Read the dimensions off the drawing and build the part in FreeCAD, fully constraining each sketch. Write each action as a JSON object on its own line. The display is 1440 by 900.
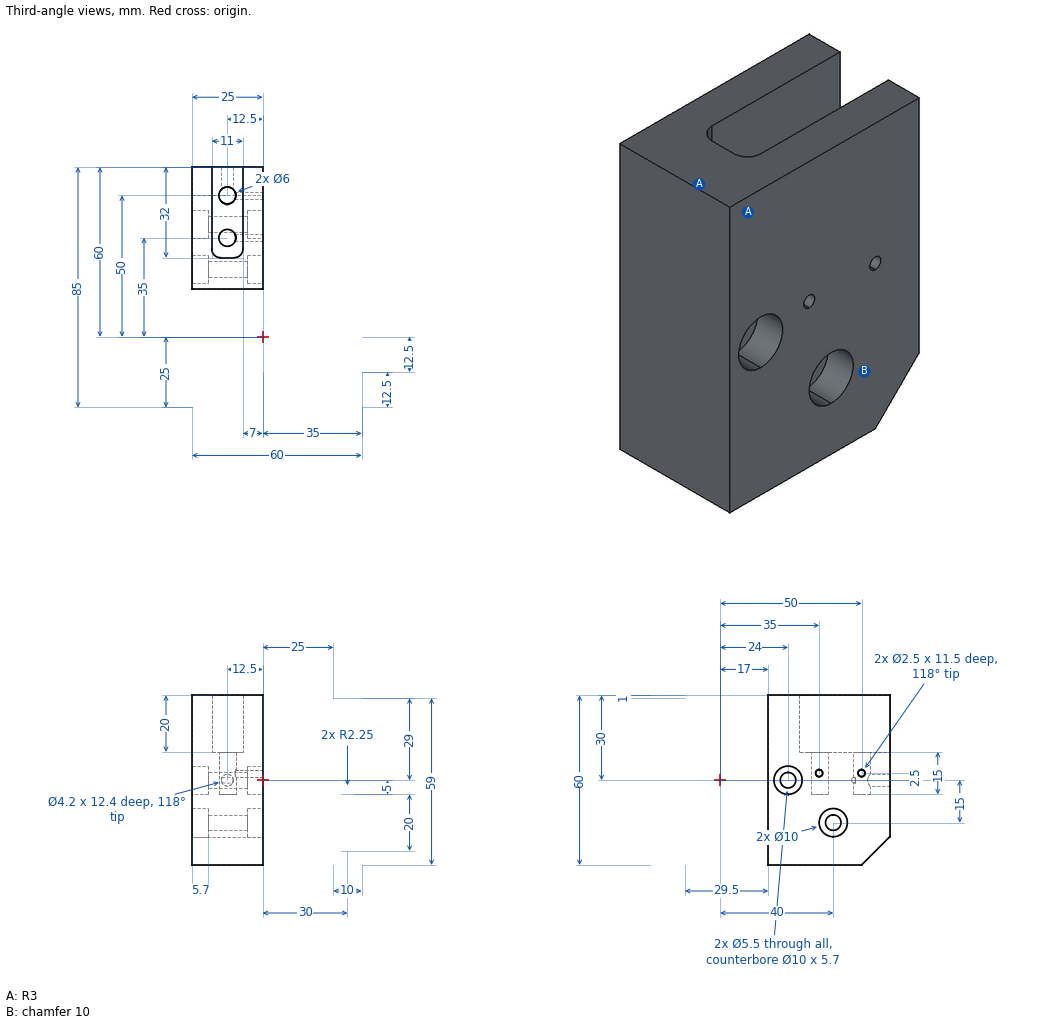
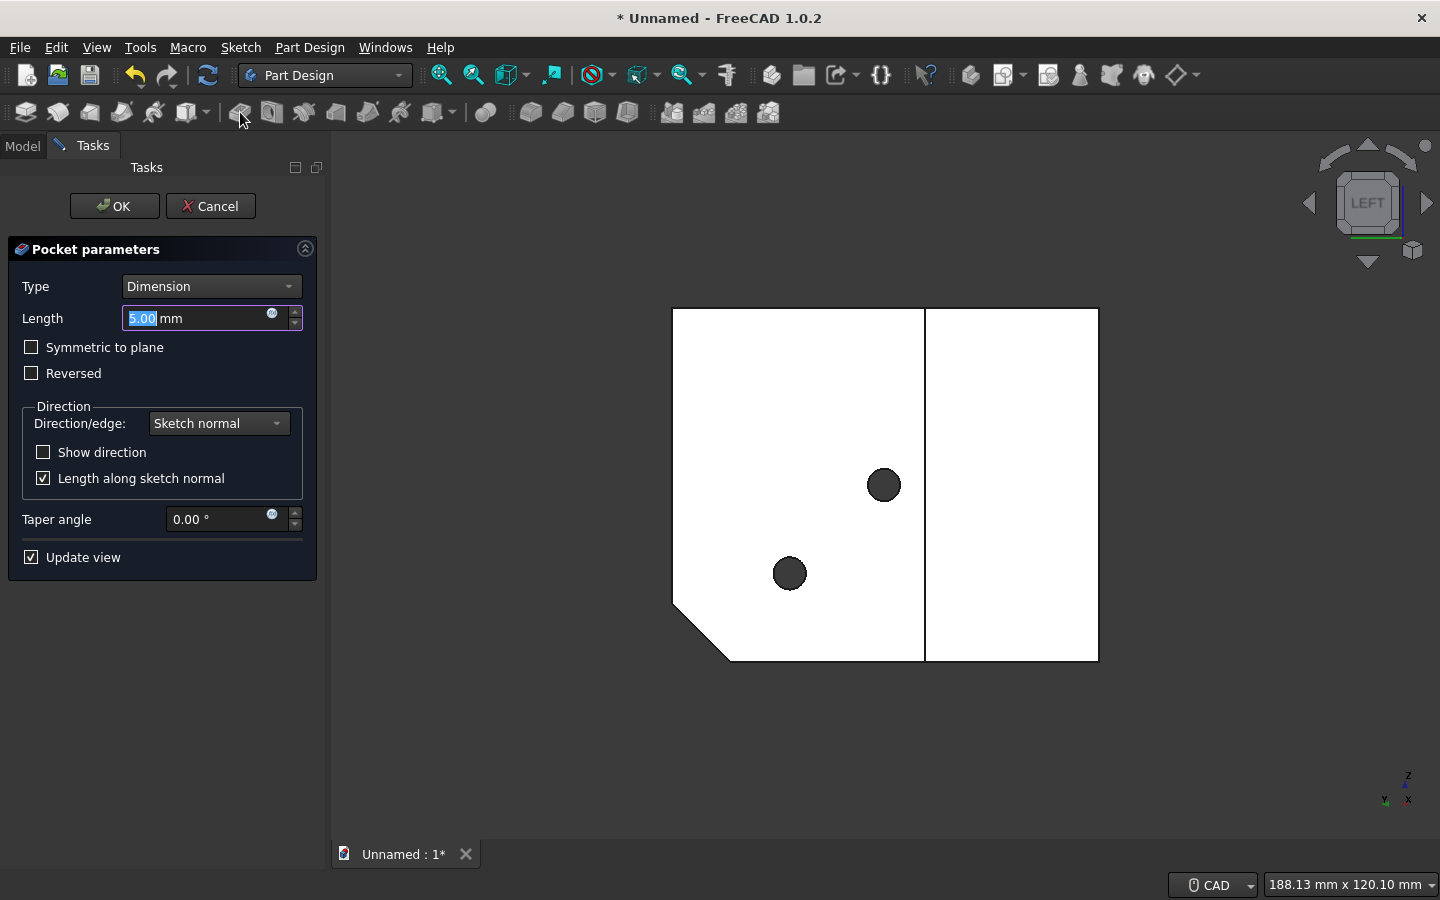
{"action": "left_click", "coordinate": [212, 286]}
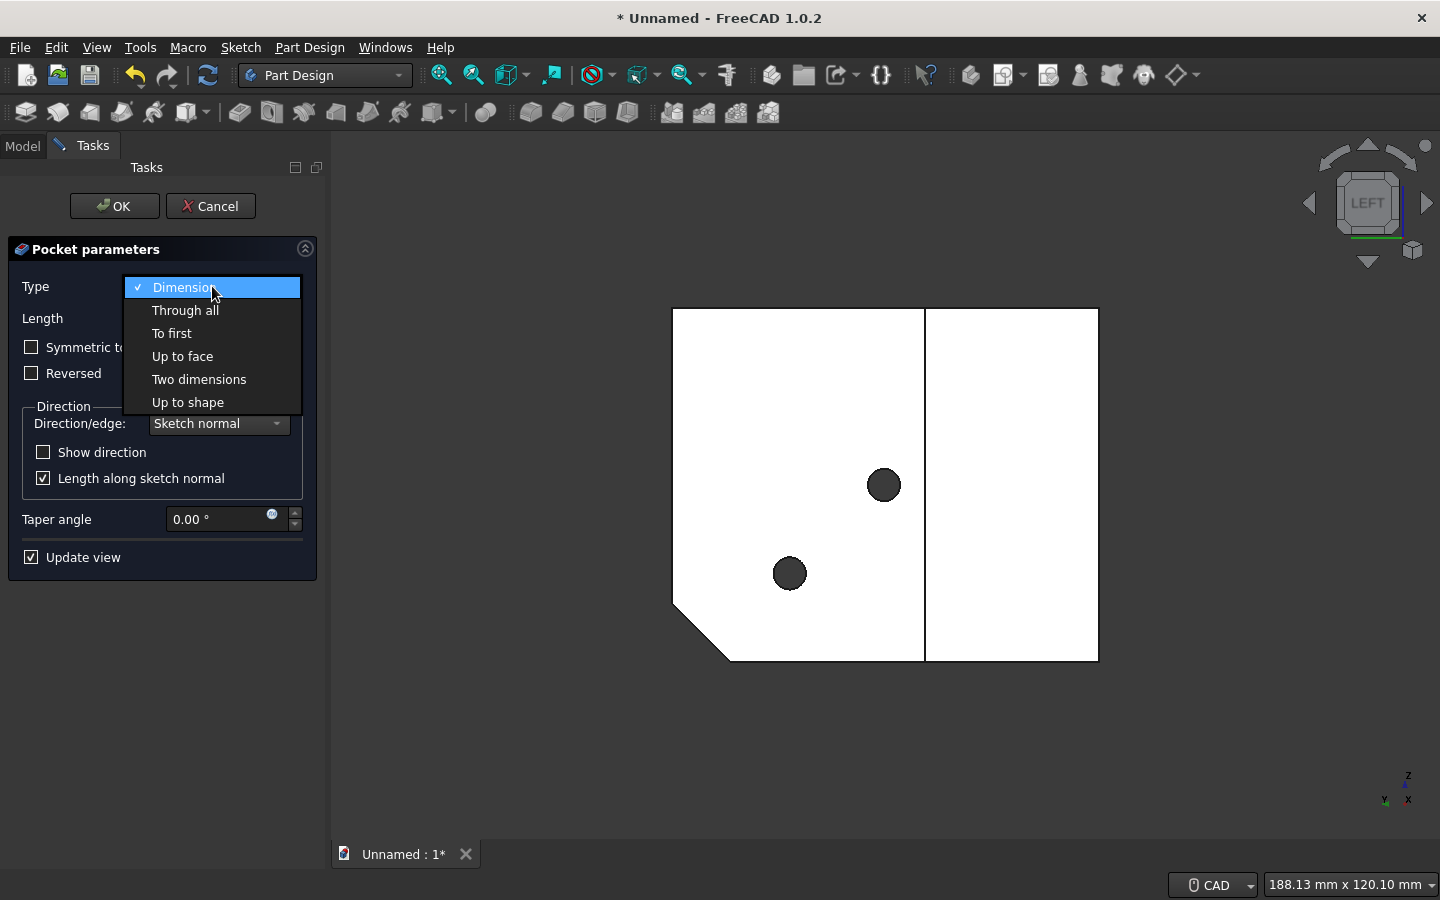
{"action": "left_click", "coordinate": [212, 310]}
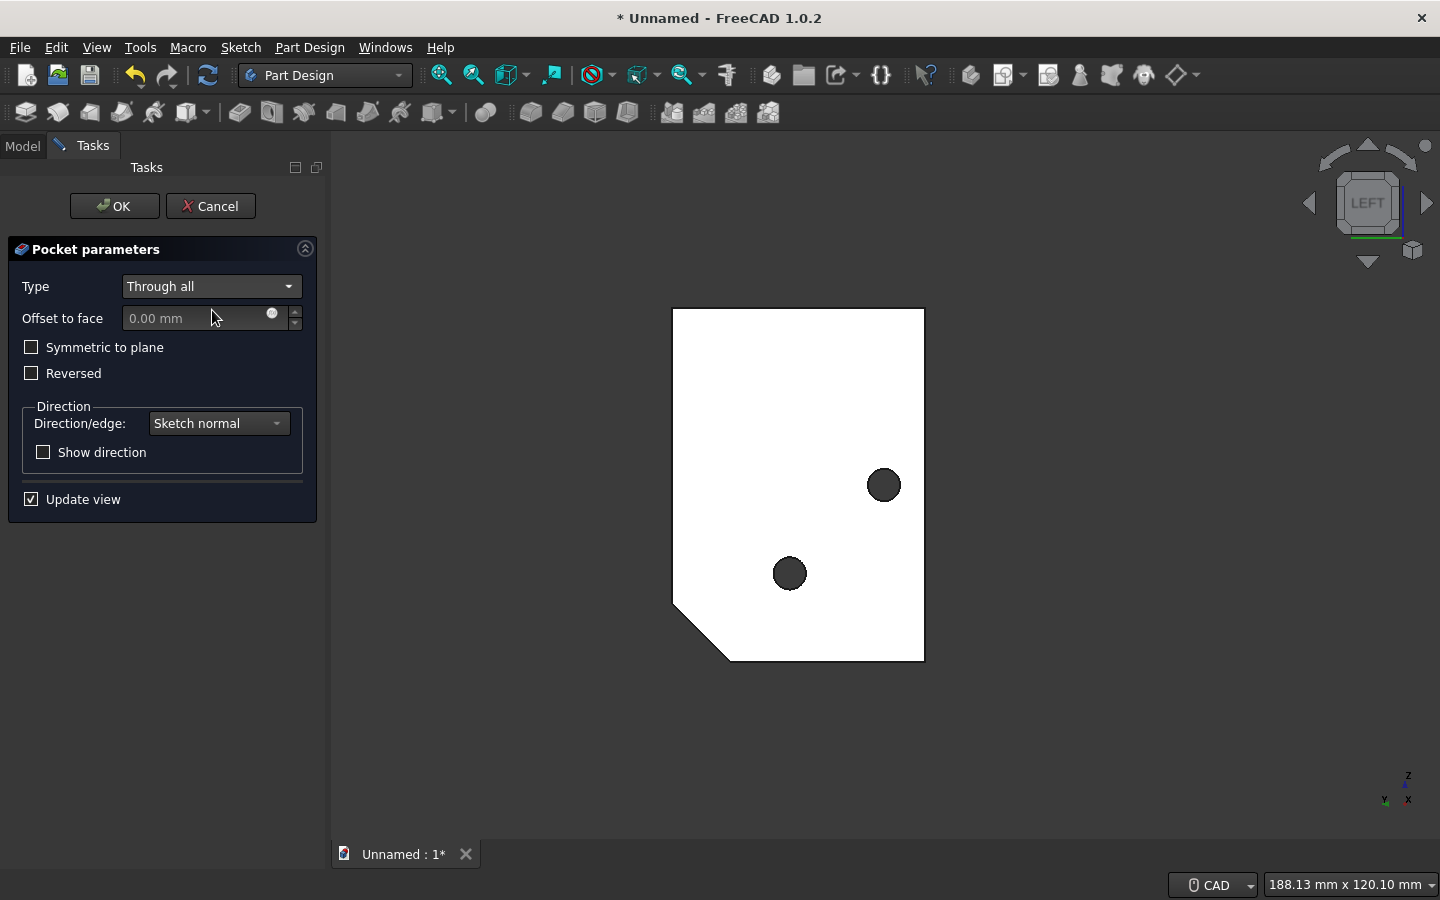
{"action": "left_click", "coordinate": [115, 206]}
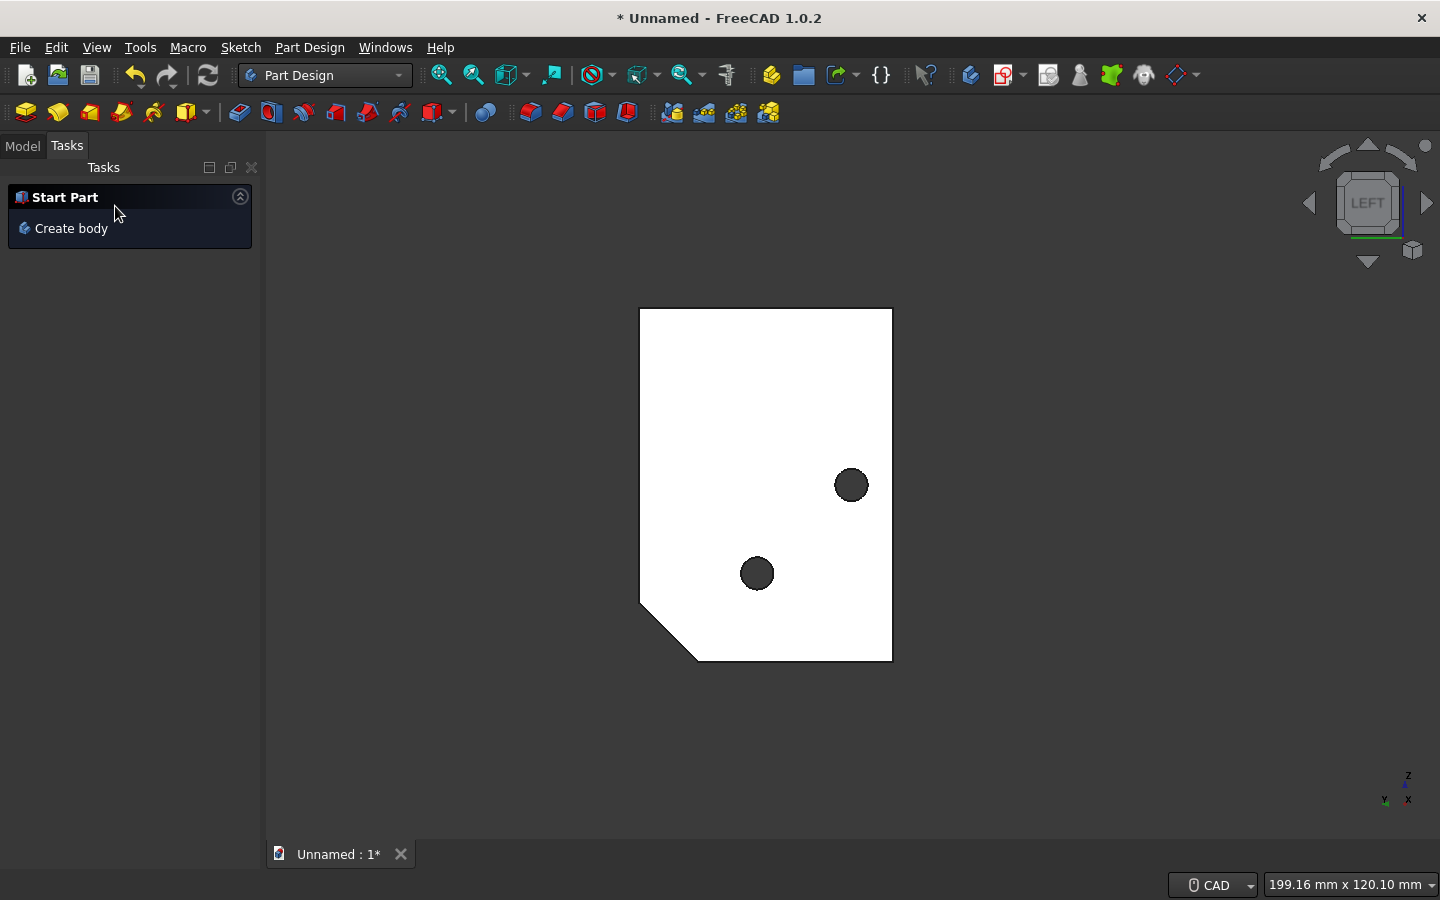
{"action": "left_click", "coordinate": [23, 145]}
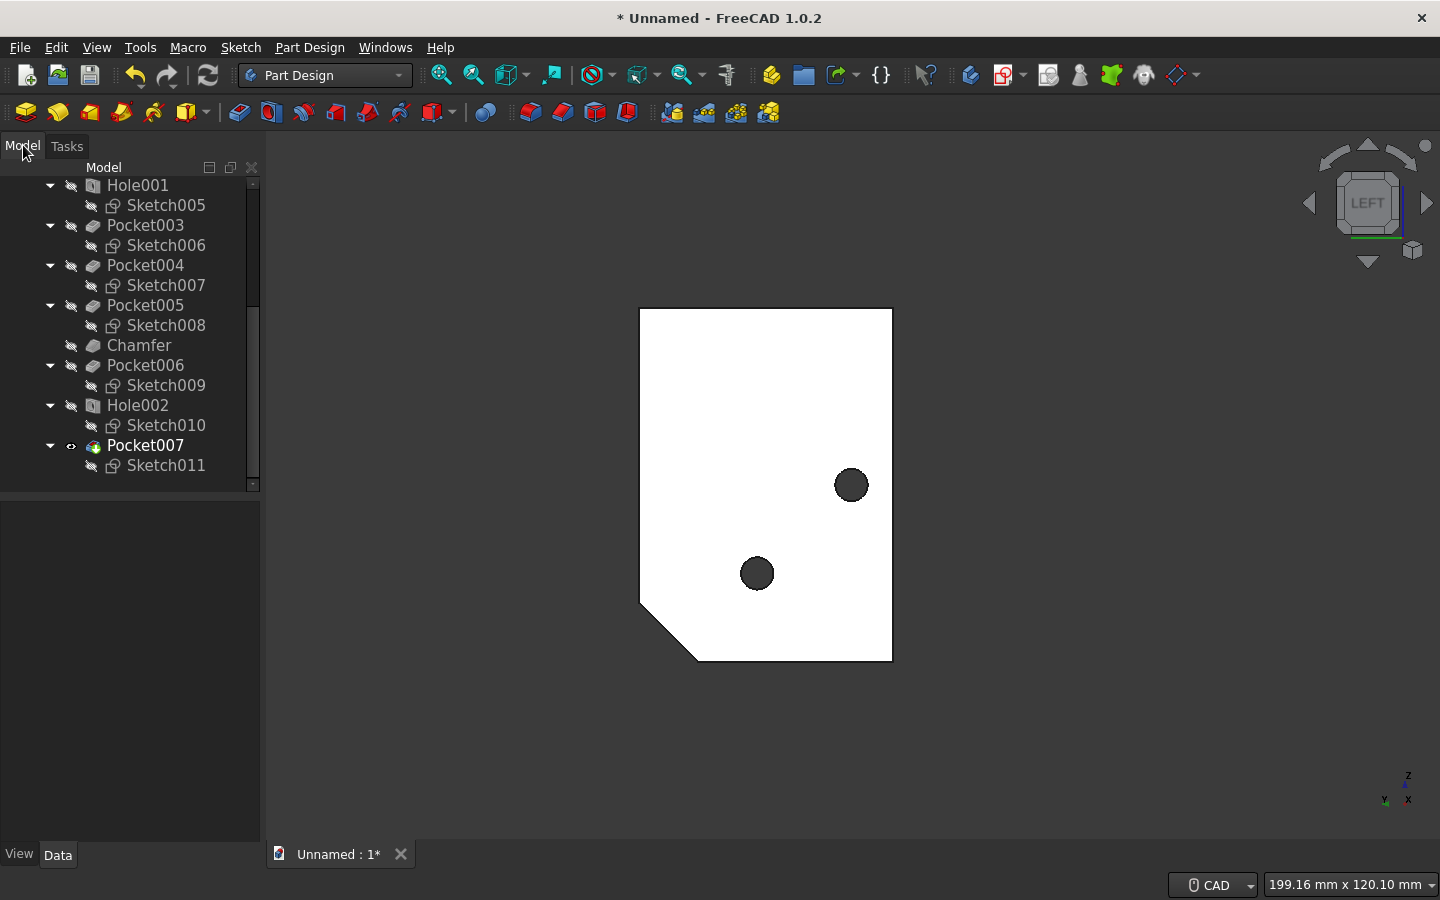
{"action": "scroll", "coordinate": [140, 321], "scroll_direction": "down", "scroll_amount": 3}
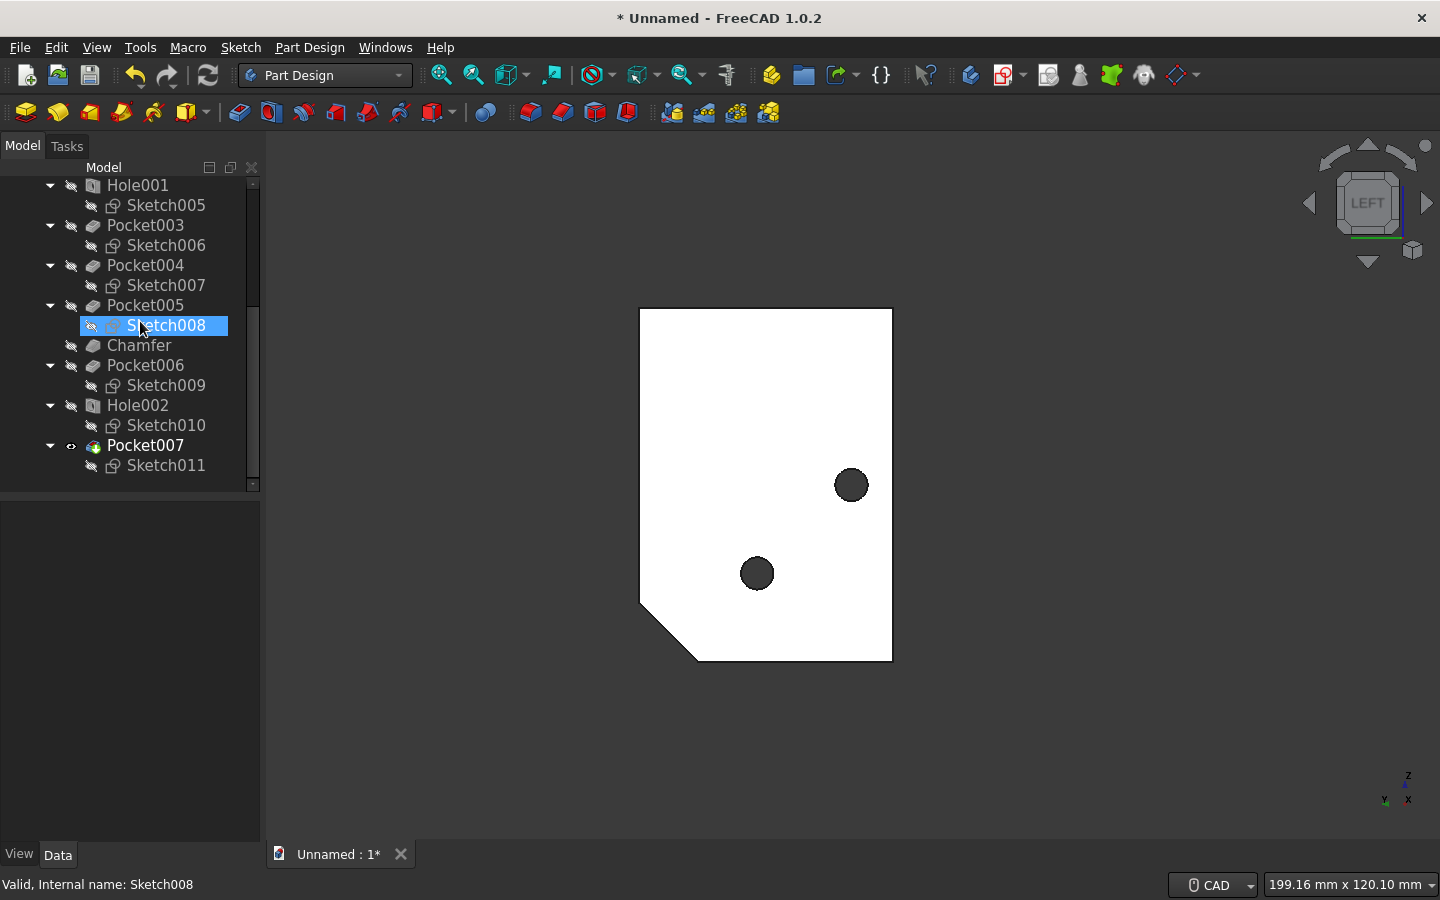
{"action": "scroll", "coordinate": [140, 321], "scroll_direction": "up", "scroll_amount": 15}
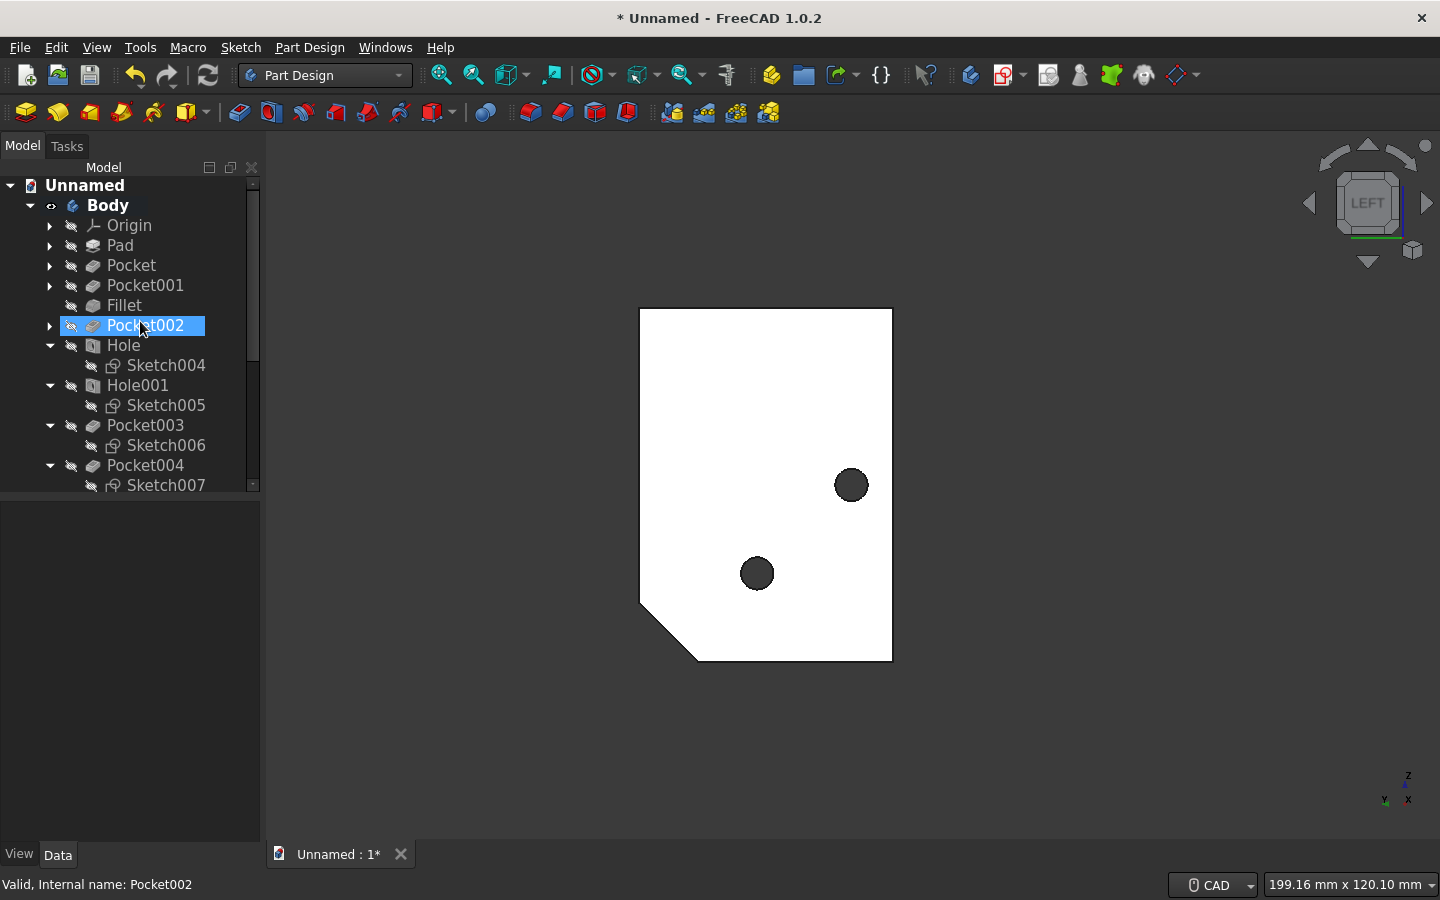
{"action": "left_click", "coordinate": [50, 226]}